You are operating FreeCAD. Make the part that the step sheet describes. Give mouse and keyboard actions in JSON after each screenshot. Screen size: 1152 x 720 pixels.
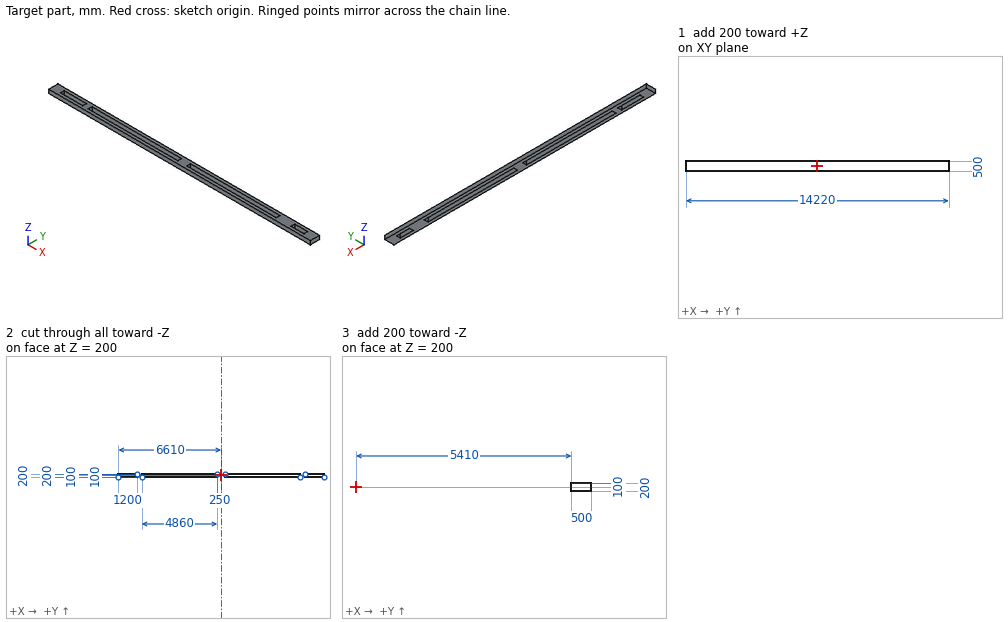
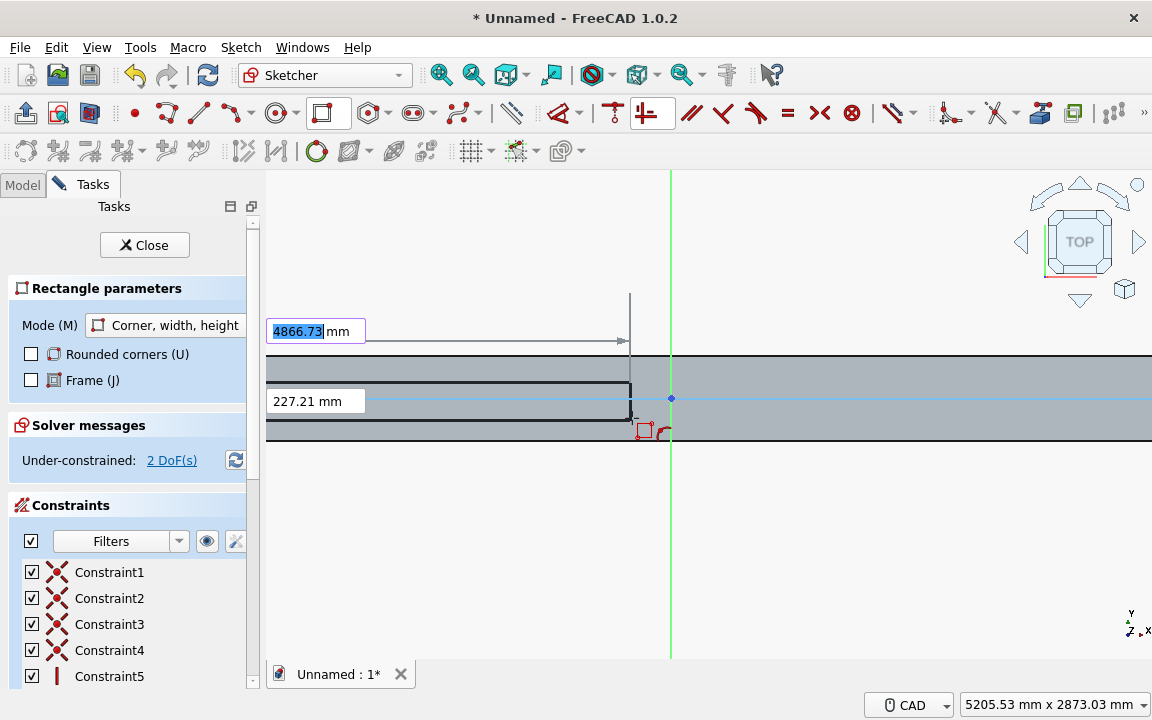
{"action": "left_click", "coordinate": [629, 416]}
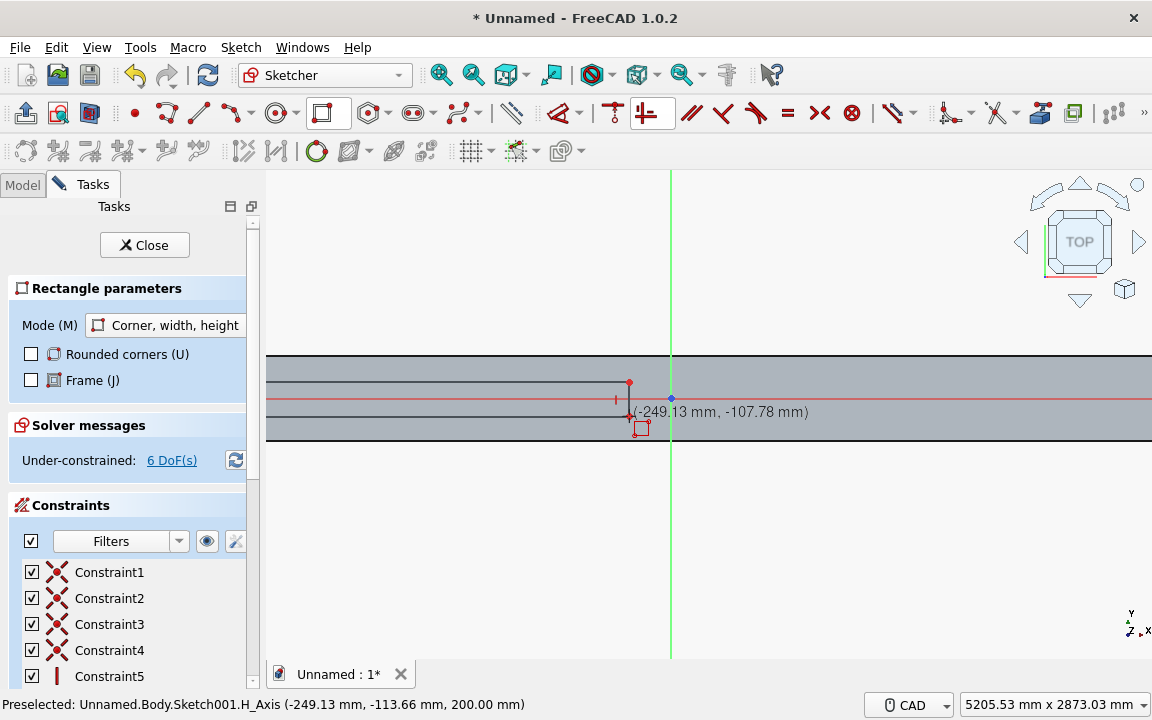
{"action": "left_click", "coordinate": [714, 382]}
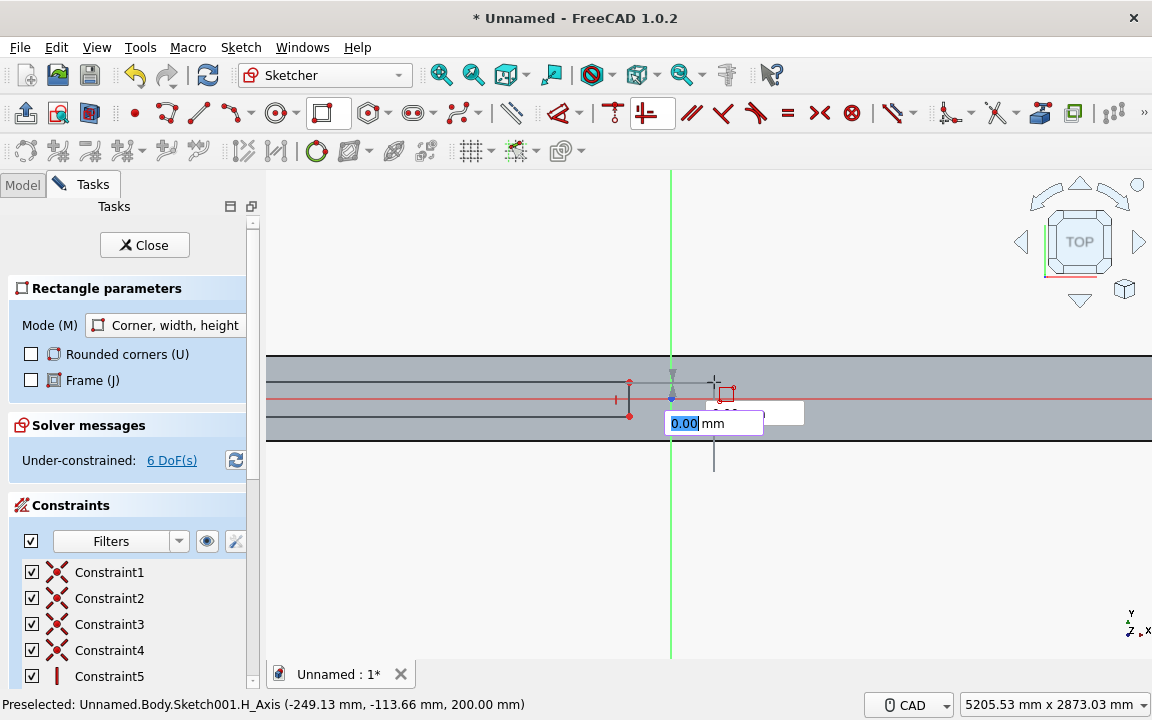
{"action": "scroll", "coordinate": [633, 419], "scroll_direction": "down", "scroll_amount": 8}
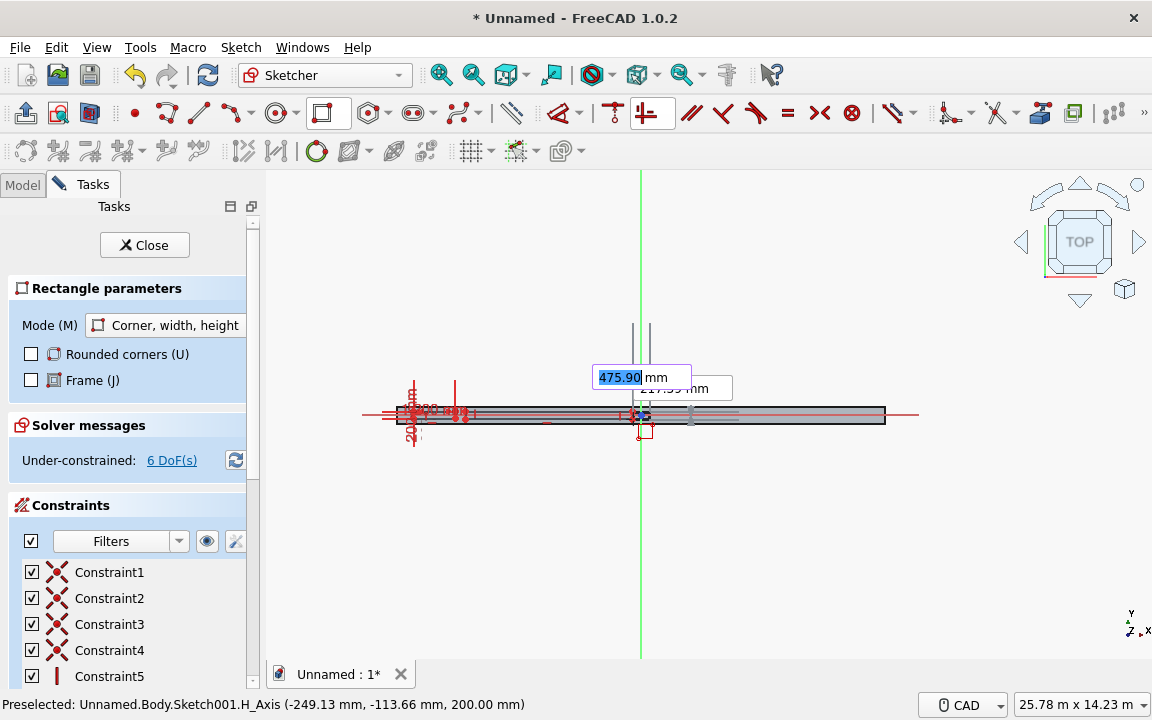
{"action": "scroll", "coordinate": [817, 419], "scroll_direction": "up", "scroll_amount": 8}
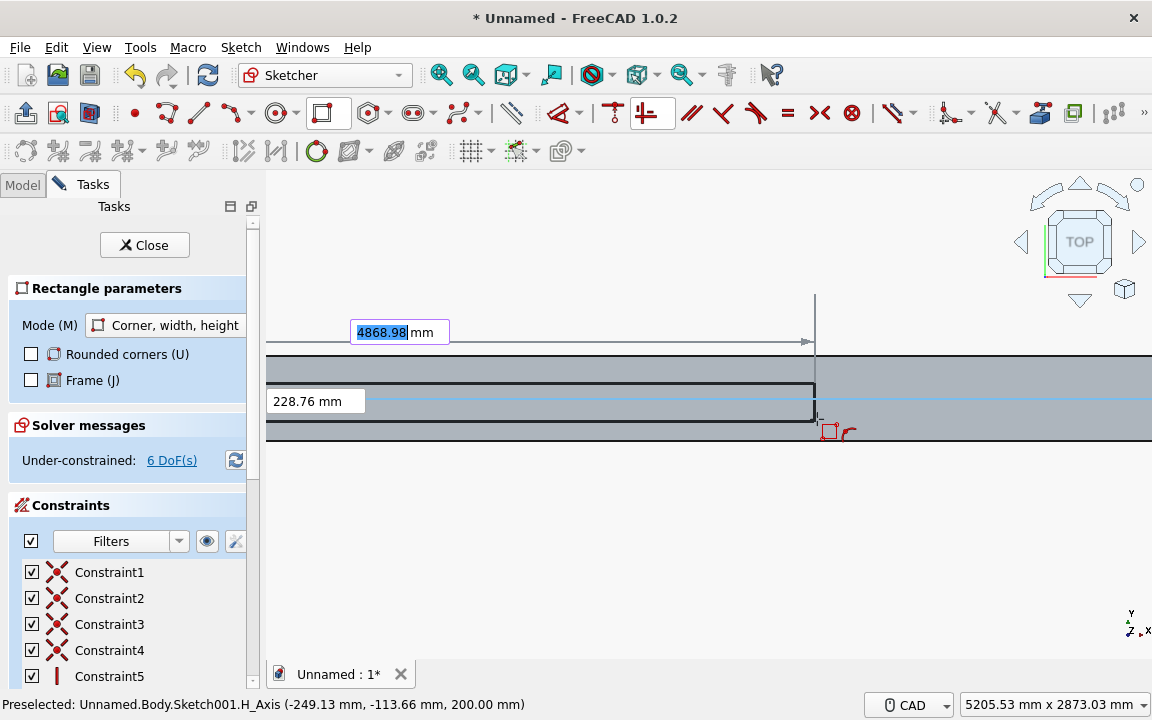
{"action": "left_click", "coordinate": [813, 416]}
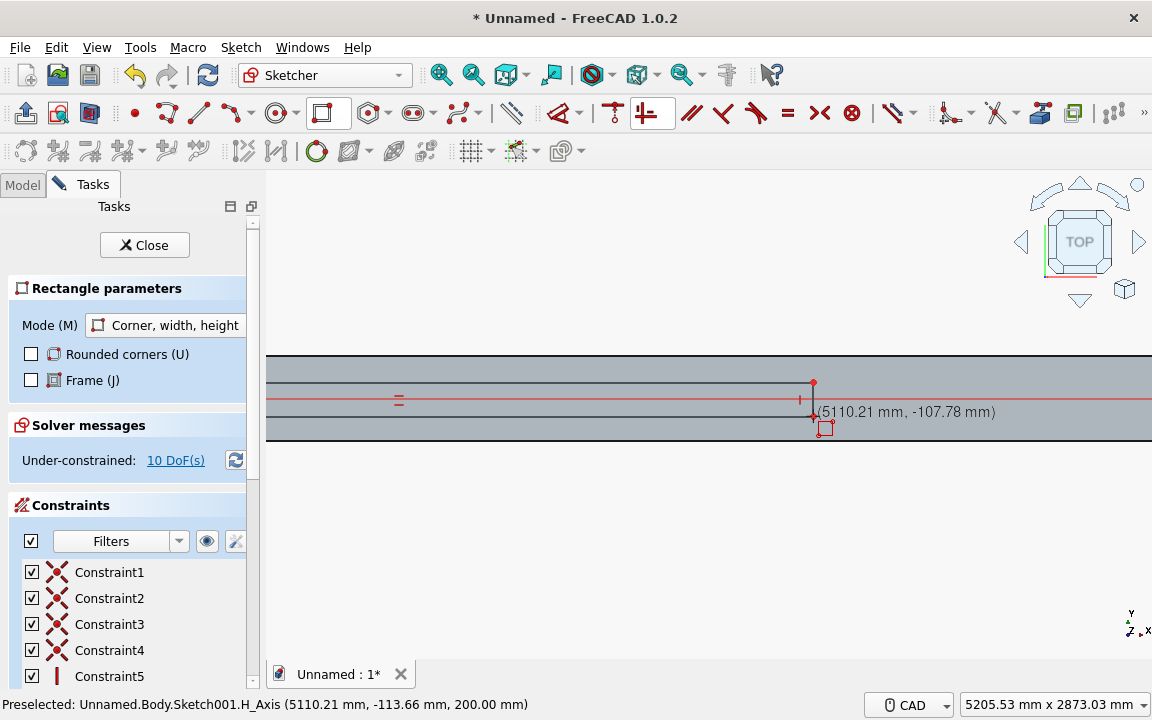
{"action": "left_click", "coordinate": [864, 382]}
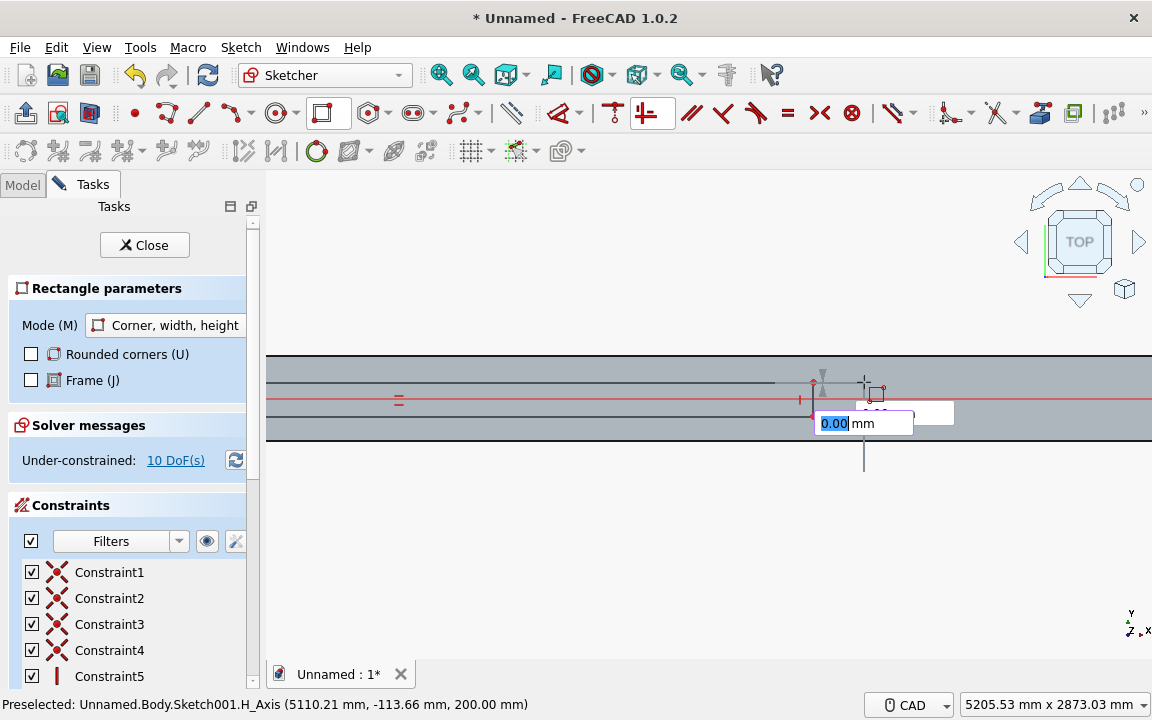
{"action": "scroll", "coordinate": [817, 419], "scroll_direction": "down", "scroll_amount": 8}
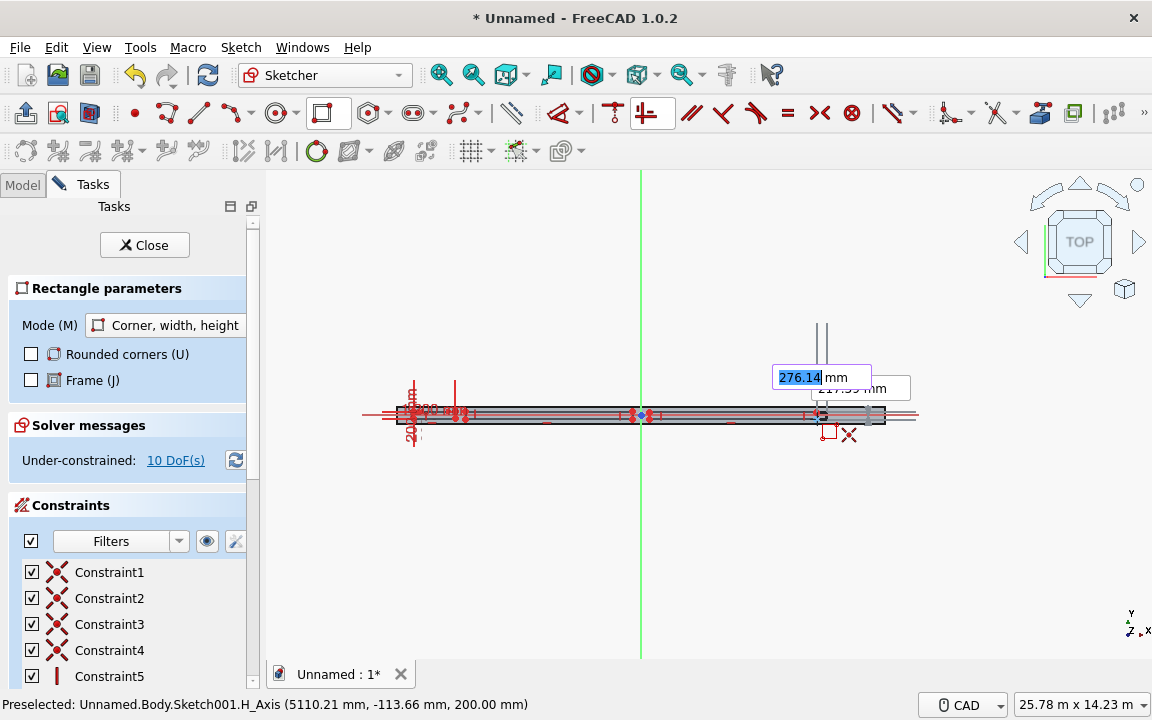
{"action": "scroll", "coordinate": [868, 419], "scroll_direction": "up", "scroll_amount": 8}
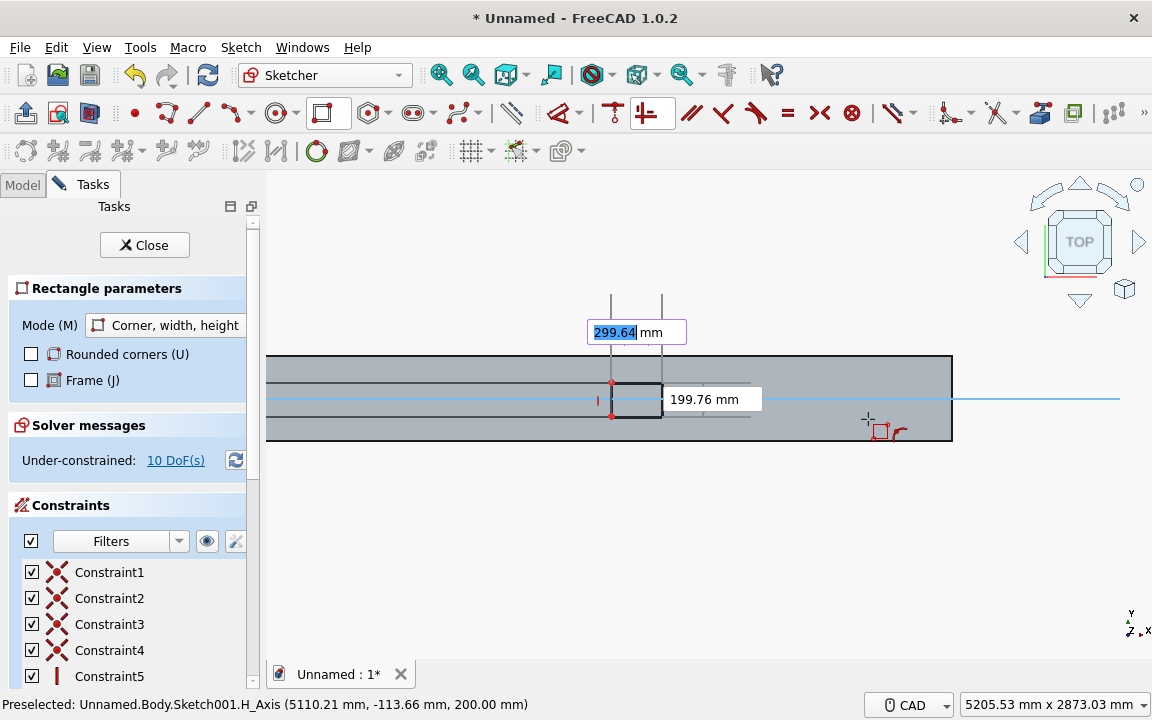
{"action": "left_click", "coordinate": [866, 416]}
{"action": "key", "text": "Escape"}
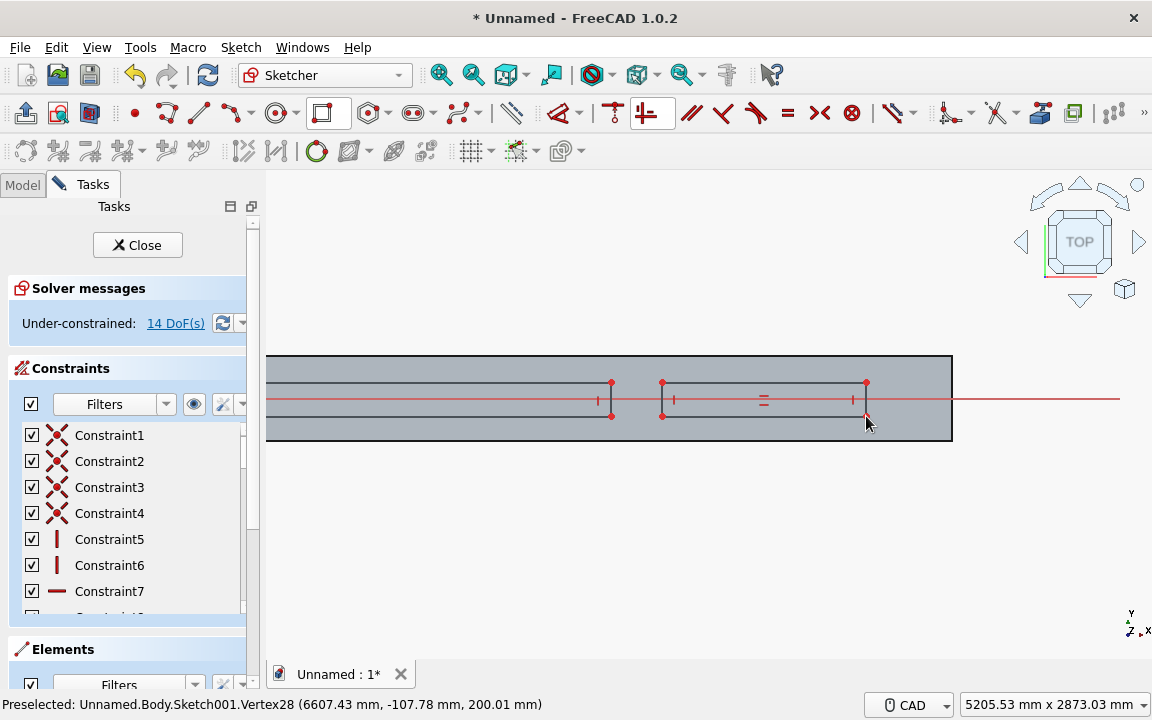
{"action": "scroll", "coordinate": [868, 419], "scroll_direction": "down", "scroll_amount": 8}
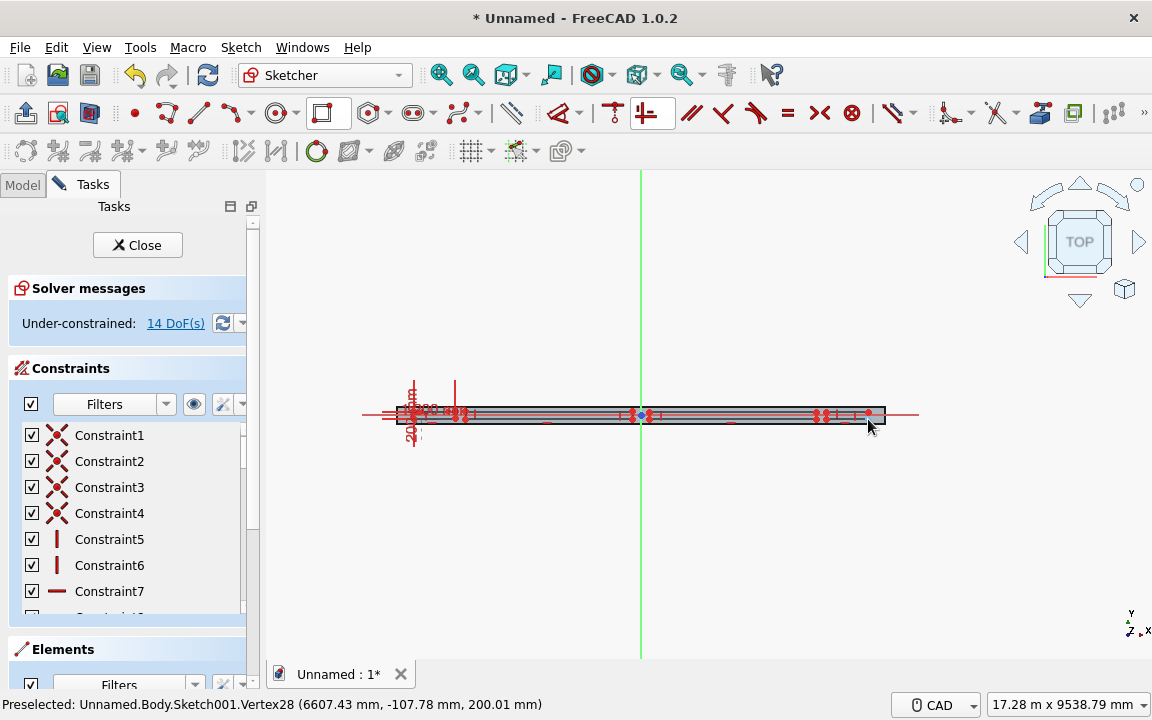
{"action": "scroll", "coordinate": [633, 412], "scroll_direction": "up", "scroll_amount": 3}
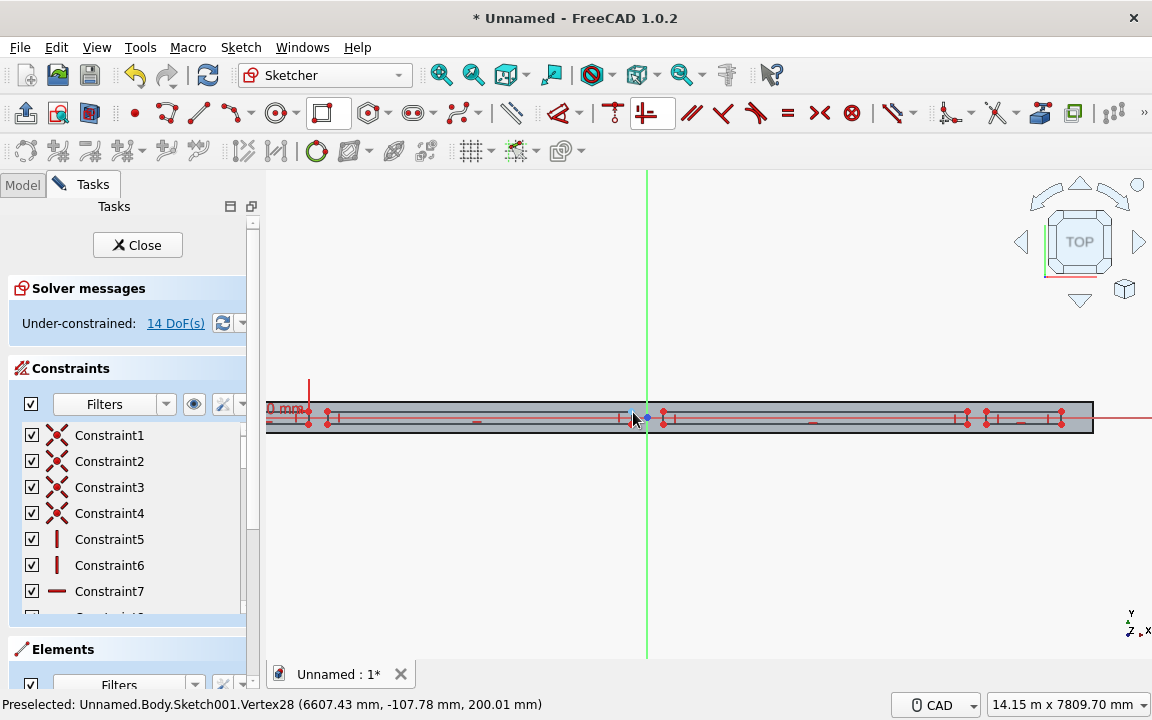
{"action": "left_click", "coordinate": [632, 412]}